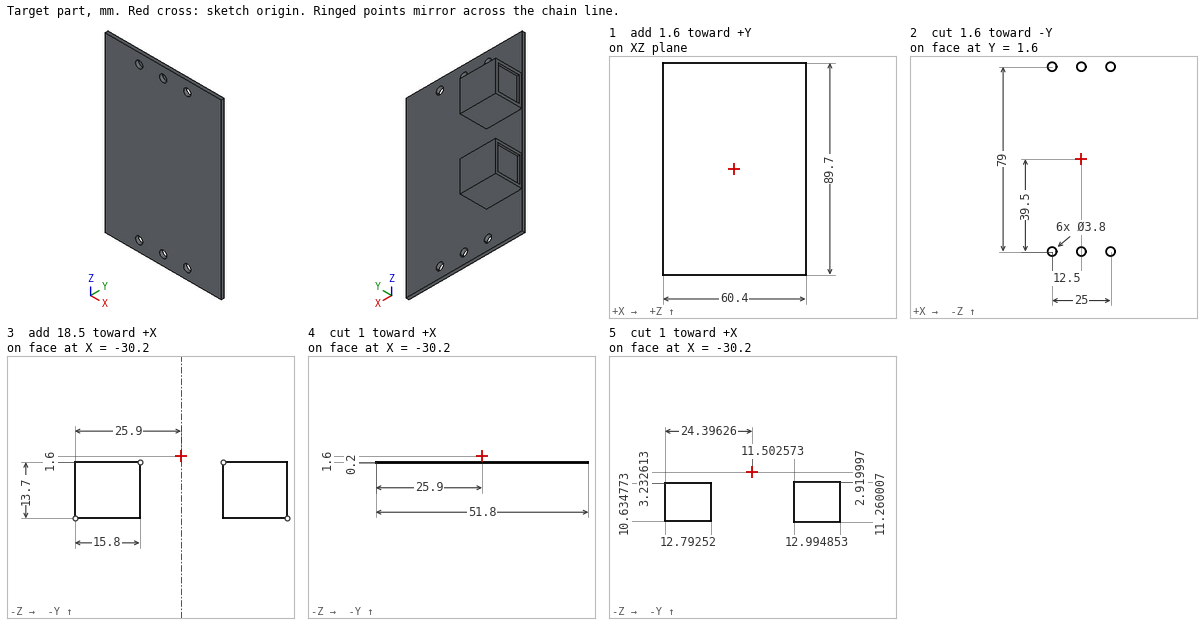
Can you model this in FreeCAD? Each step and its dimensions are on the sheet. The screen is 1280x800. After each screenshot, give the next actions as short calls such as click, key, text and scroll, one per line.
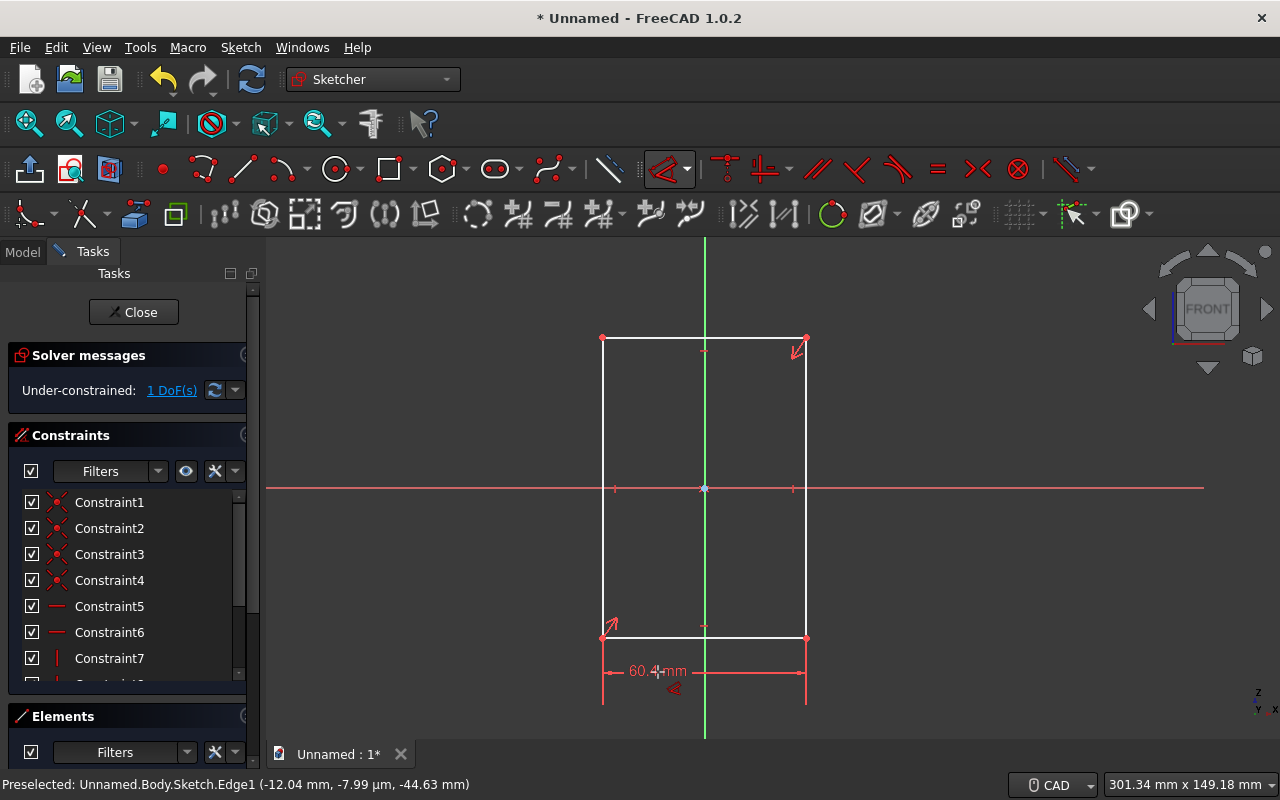
click(806, 548)
click(840, 419)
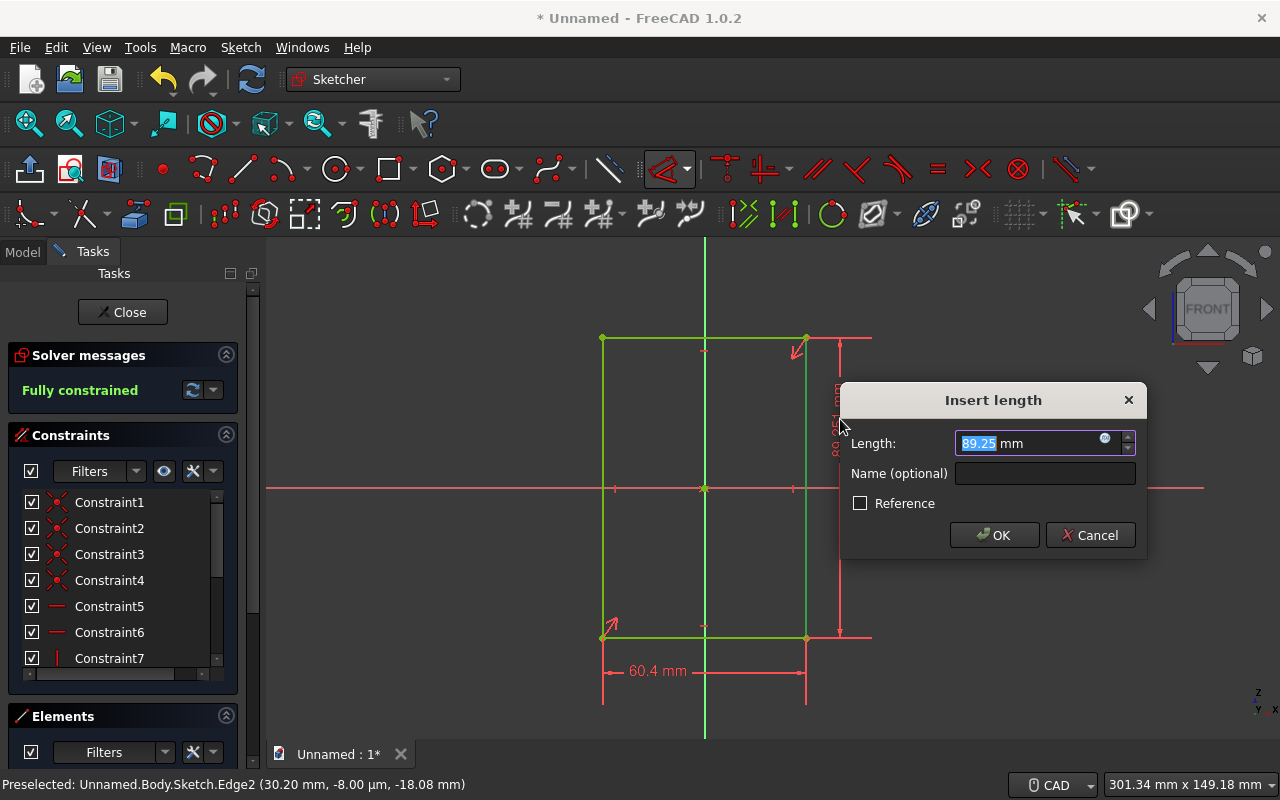
text(89.7)
key(Return)
key(Escape)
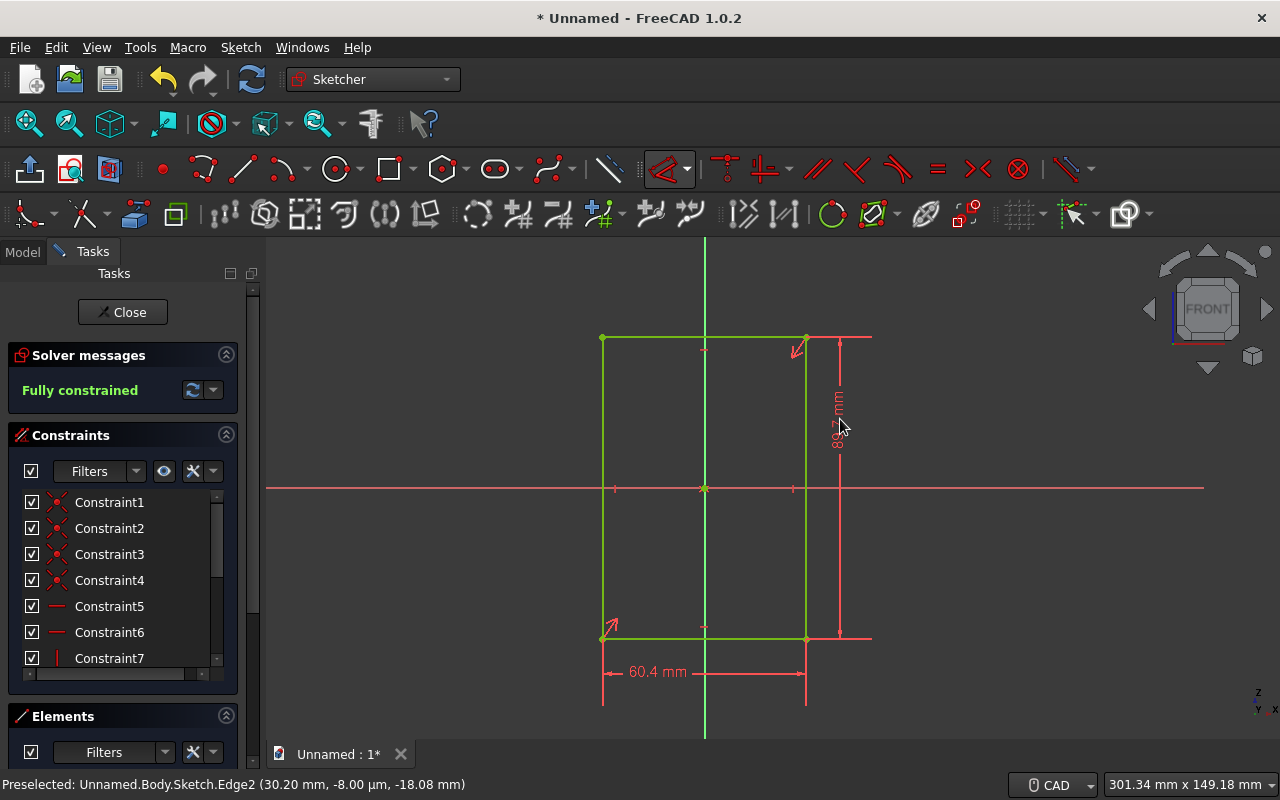
click(123, 312)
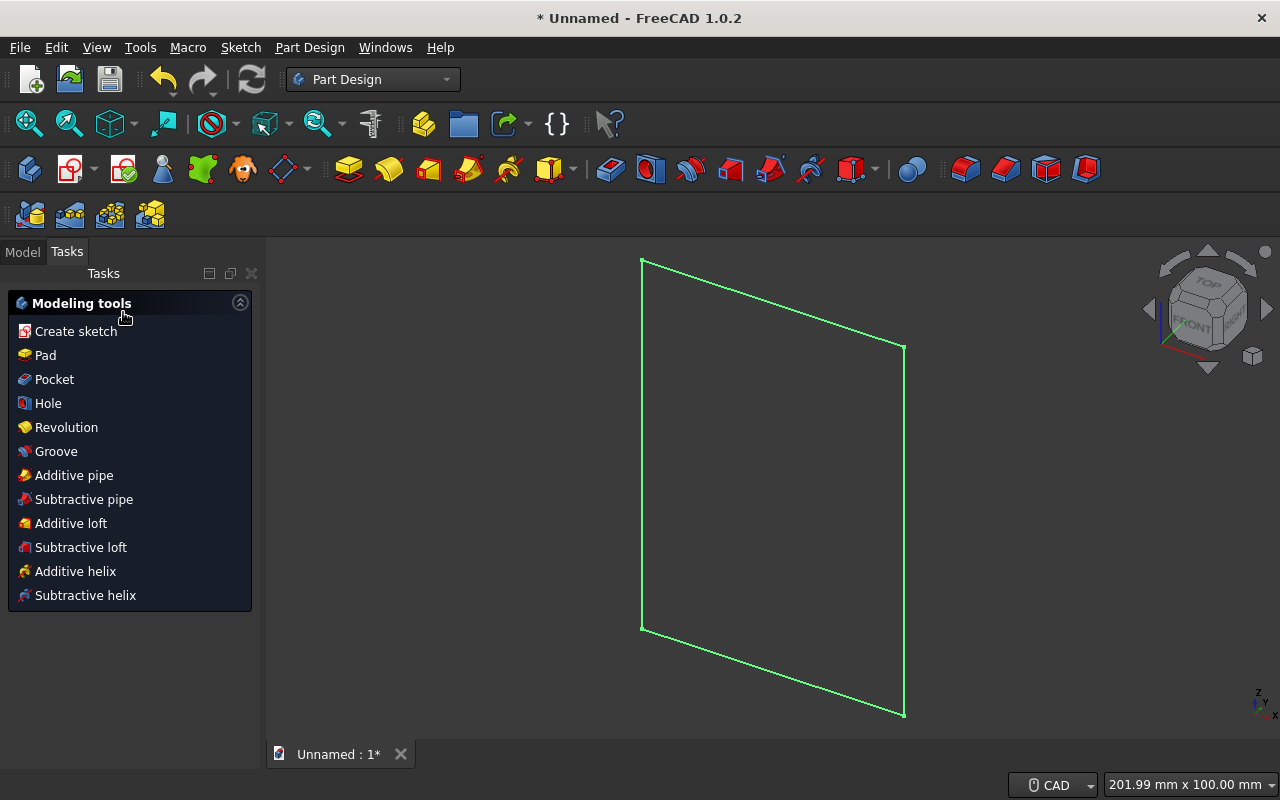
click(350, 170)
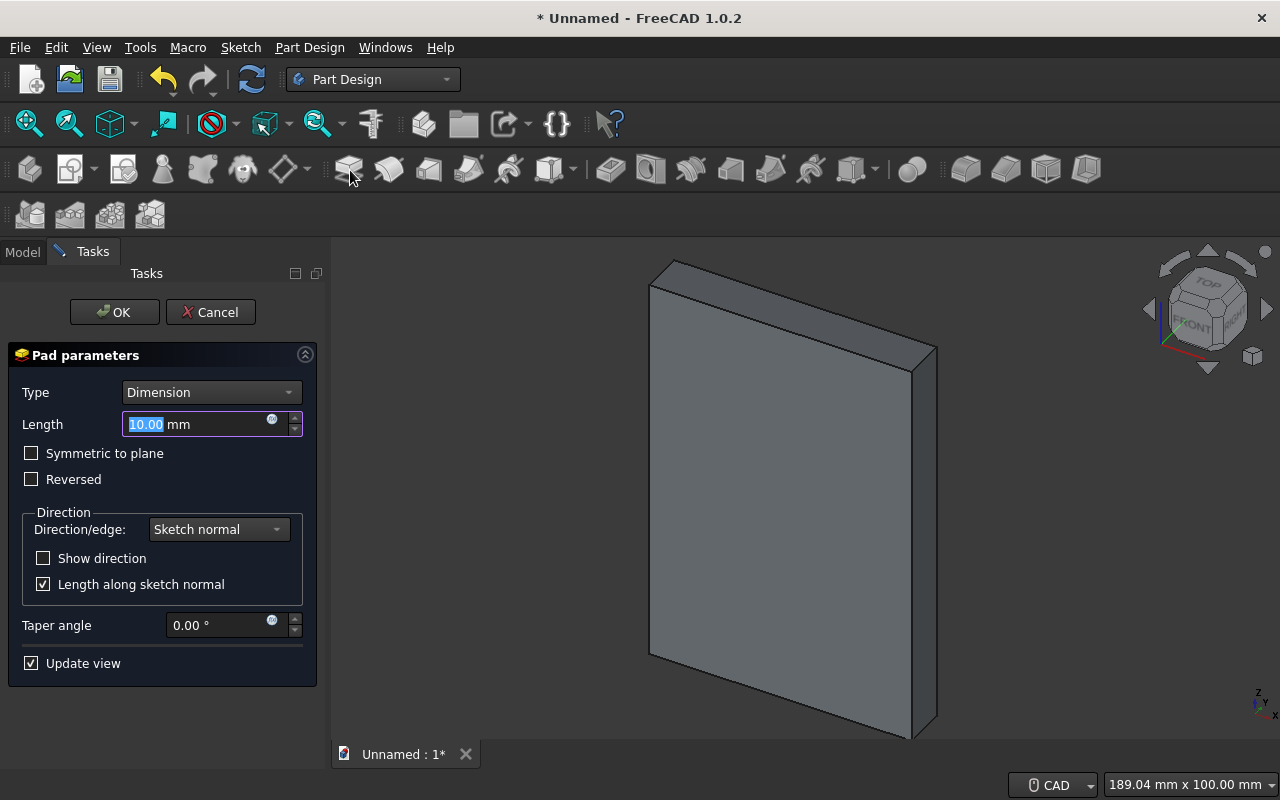
text(1.6)
key(Tab)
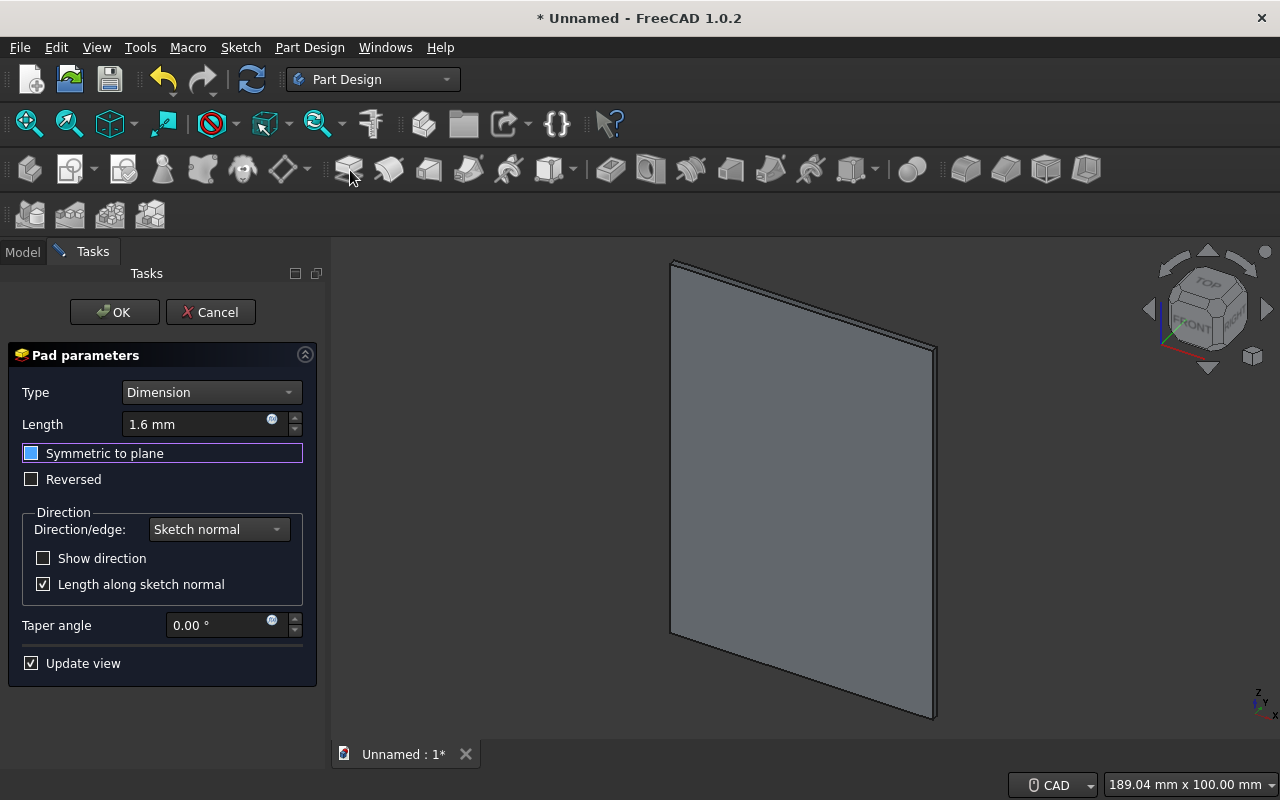
click(30, 479)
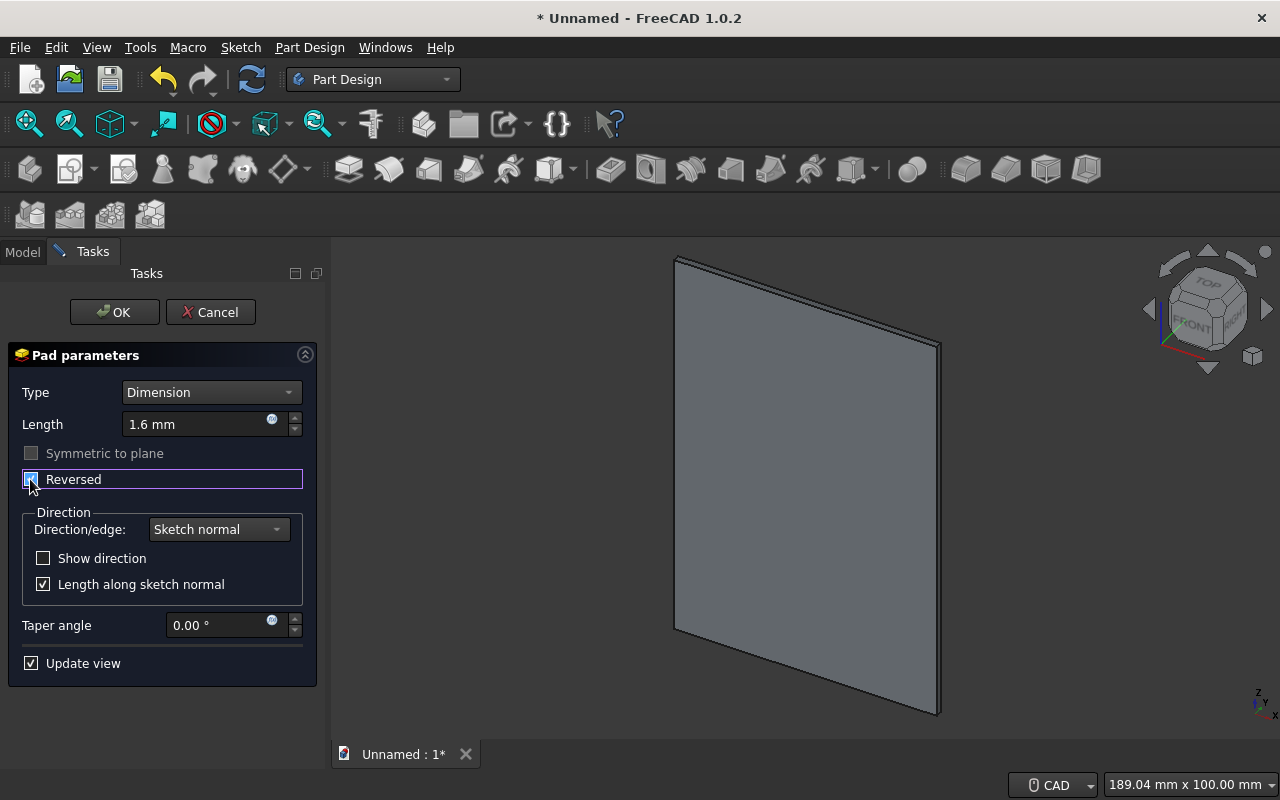
click(115, 312)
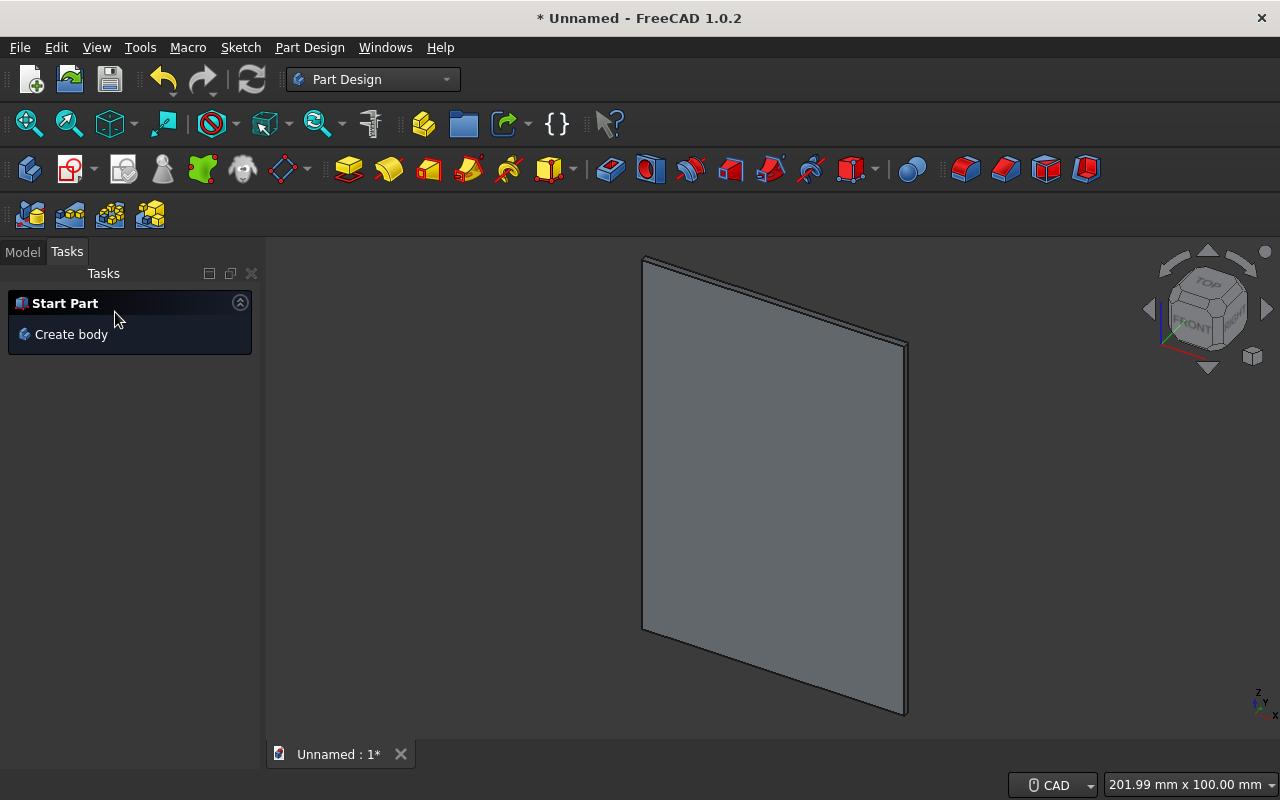
key(4)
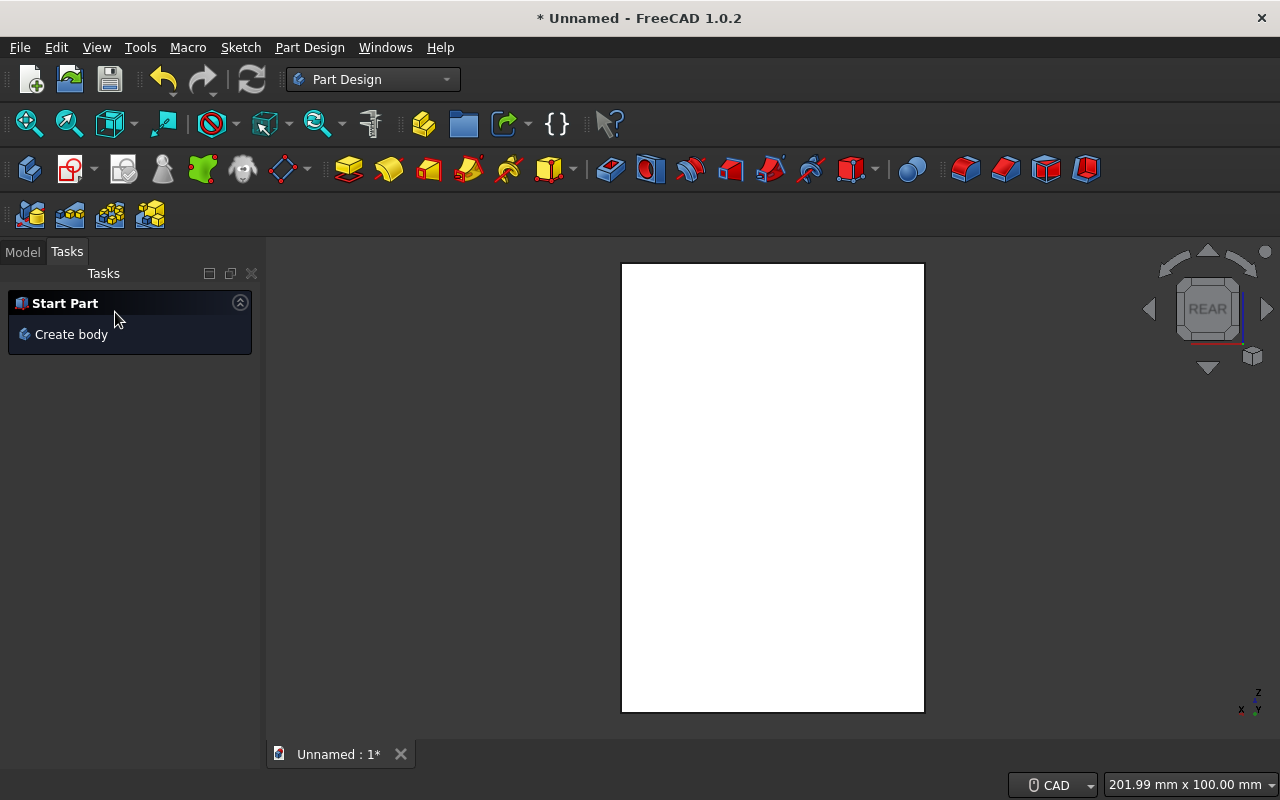
click(773, 423)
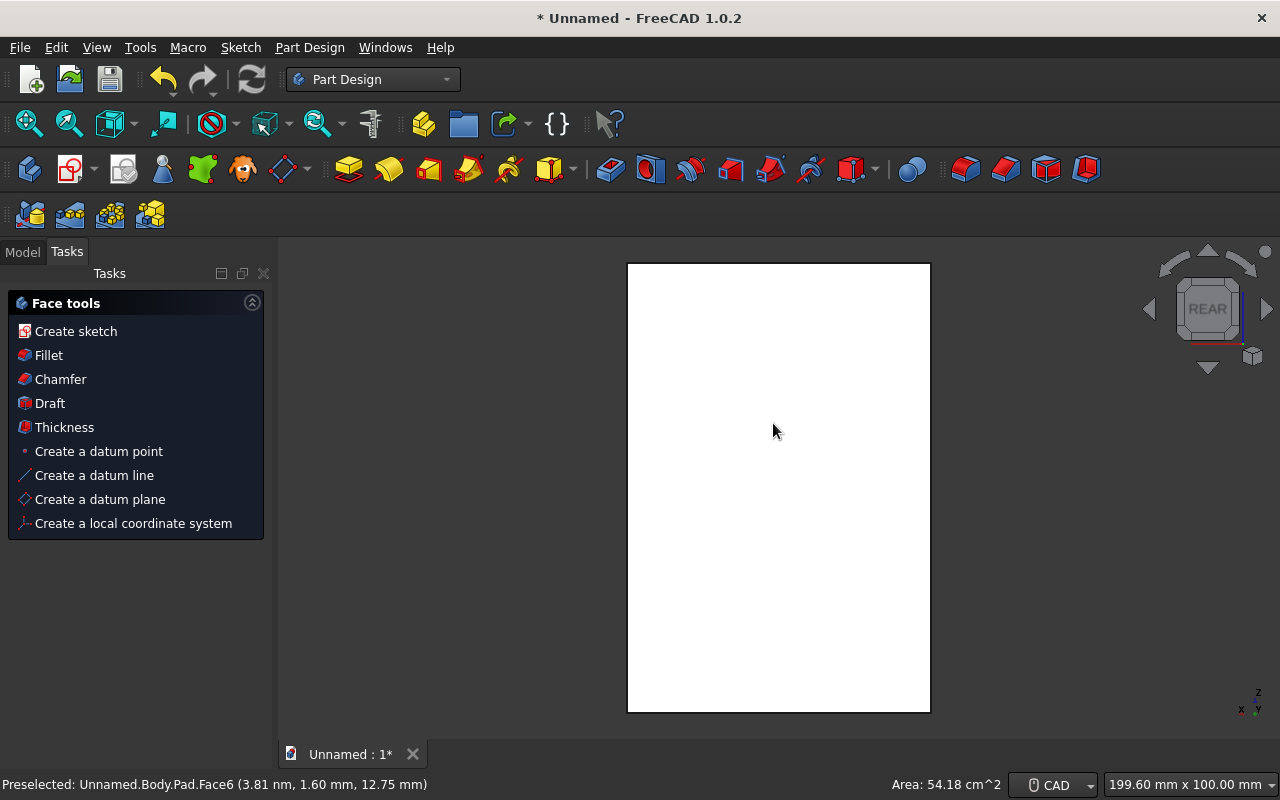
click(70, 170)